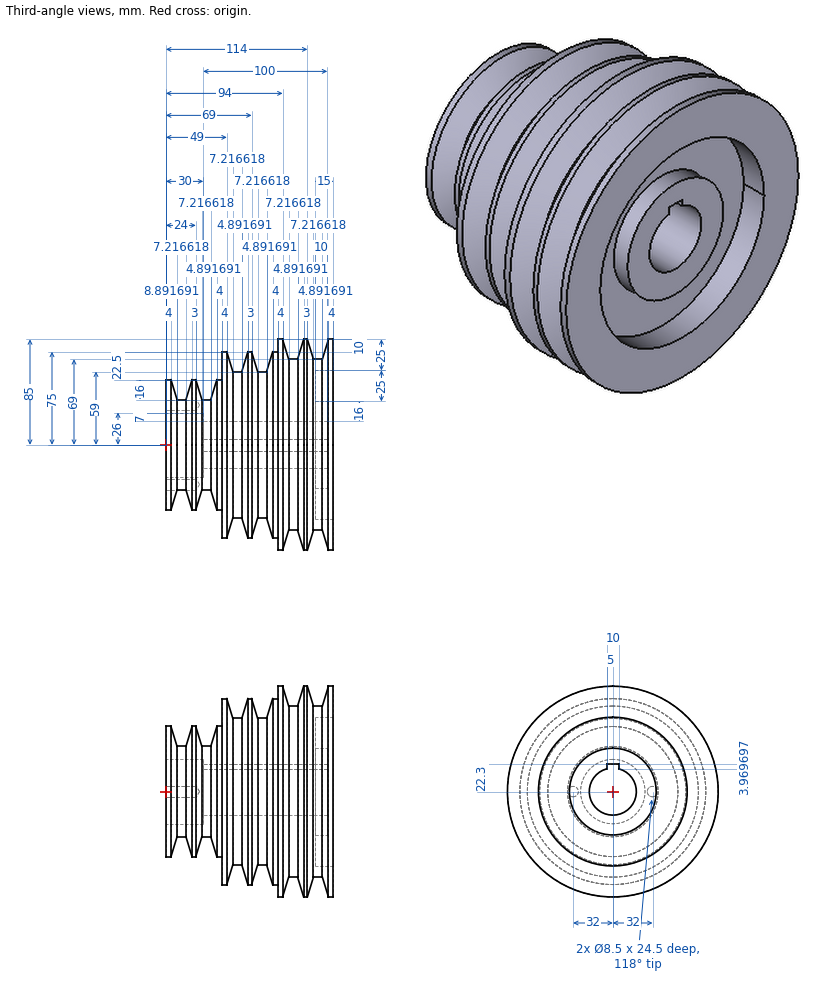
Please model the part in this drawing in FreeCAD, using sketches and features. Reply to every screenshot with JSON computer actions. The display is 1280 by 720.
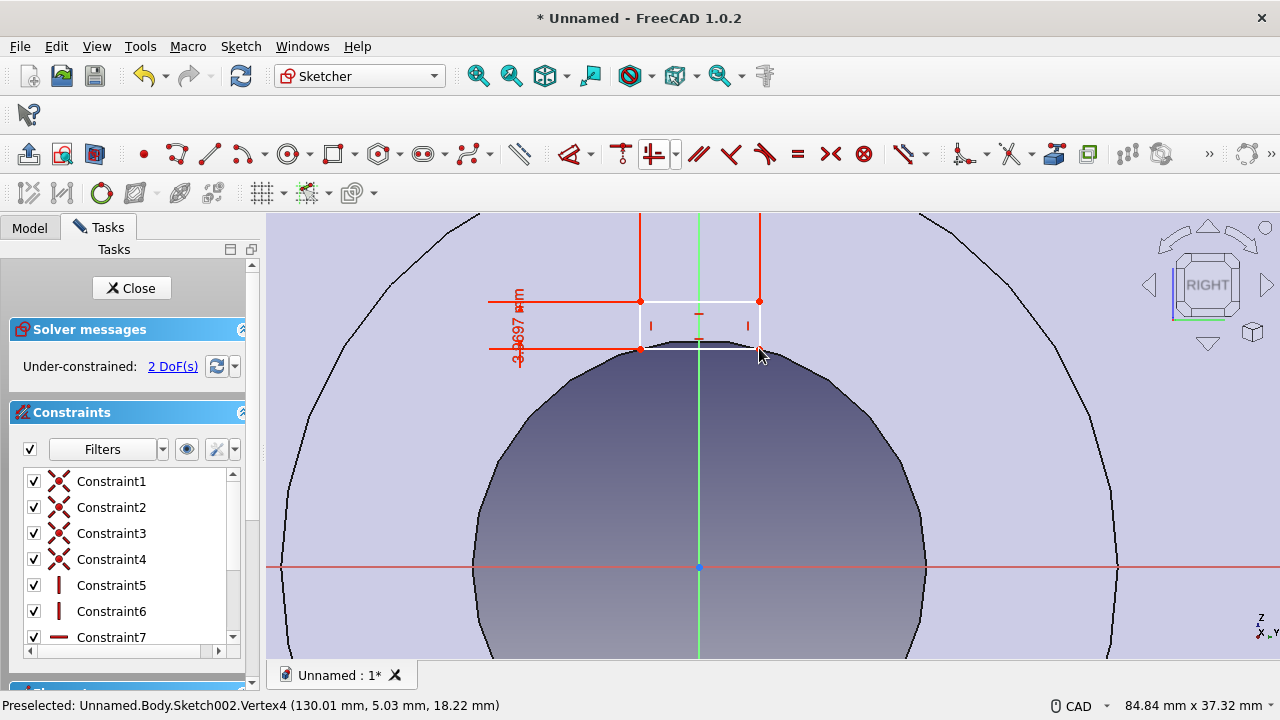
{"action": "left_click", "coordinate": [568, 154]}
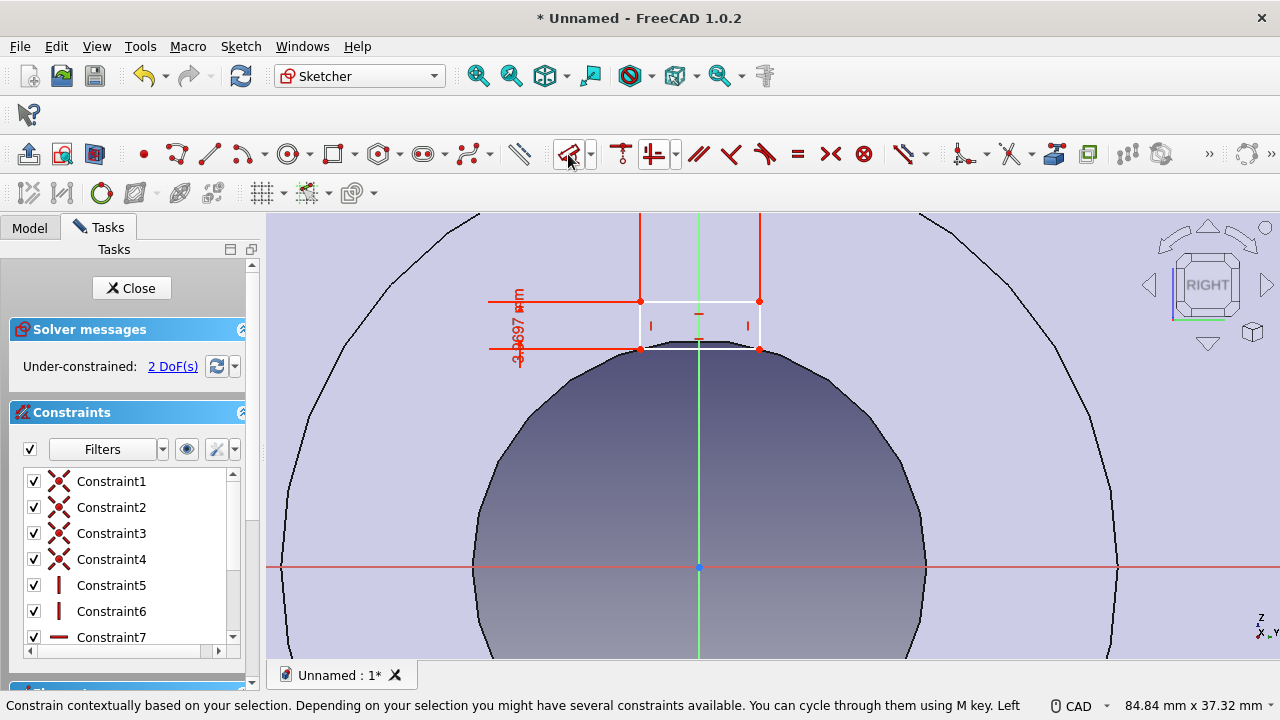
{"action": "left_click", "coordinate": [640, 302]}
{"action": "left_click", "coordinate": [670, 601]}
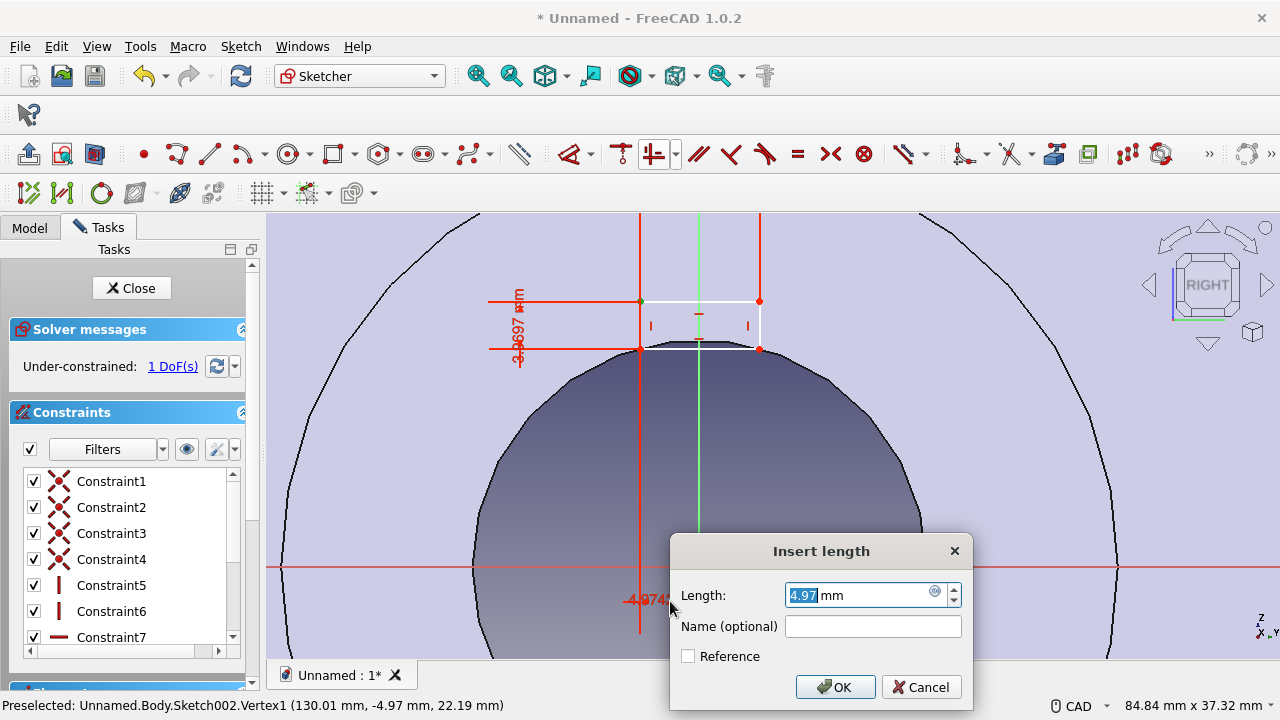
{"action": "type", "text": "5"}
{"action": "key", "text": "Return"}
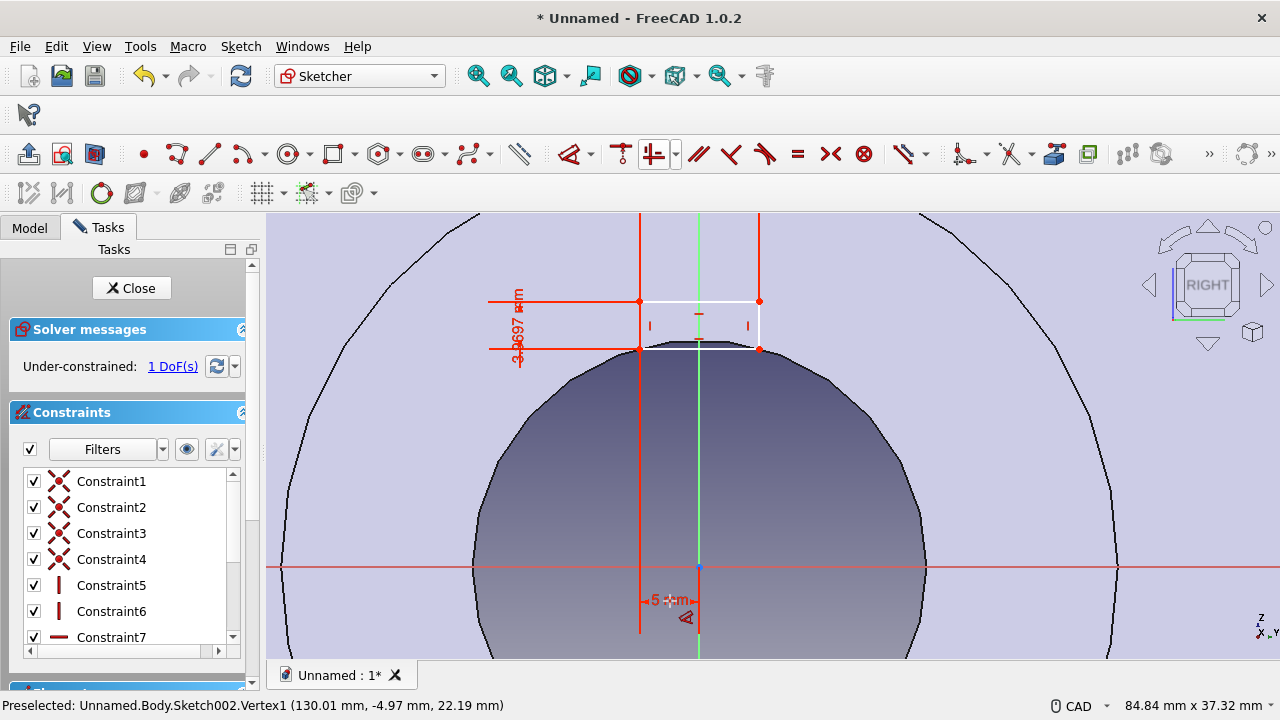
{"action": "left_click", "coordinate": [640, 302]}
{"action": "left_click", "coordinate": [606, 435]}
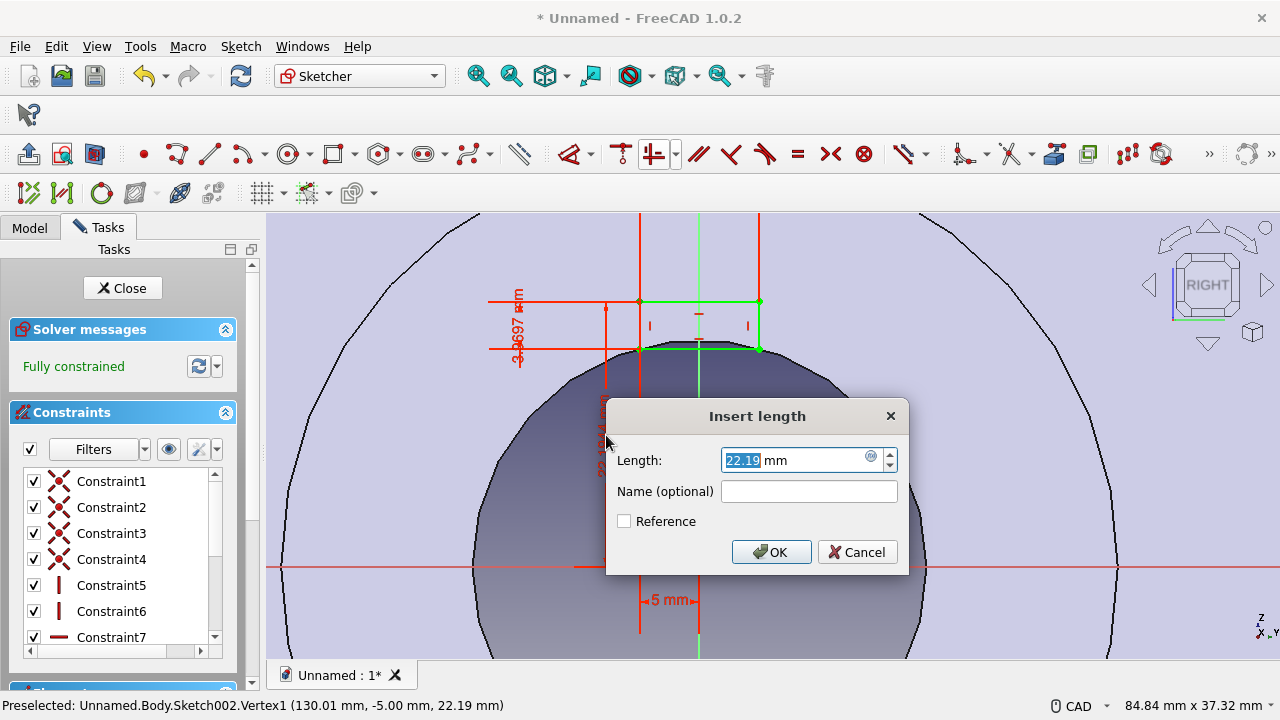
{"action": "type", "text": "22.3"}
{"action": "key", "text": "Return"}
{"action": "key", "text": "Escape"}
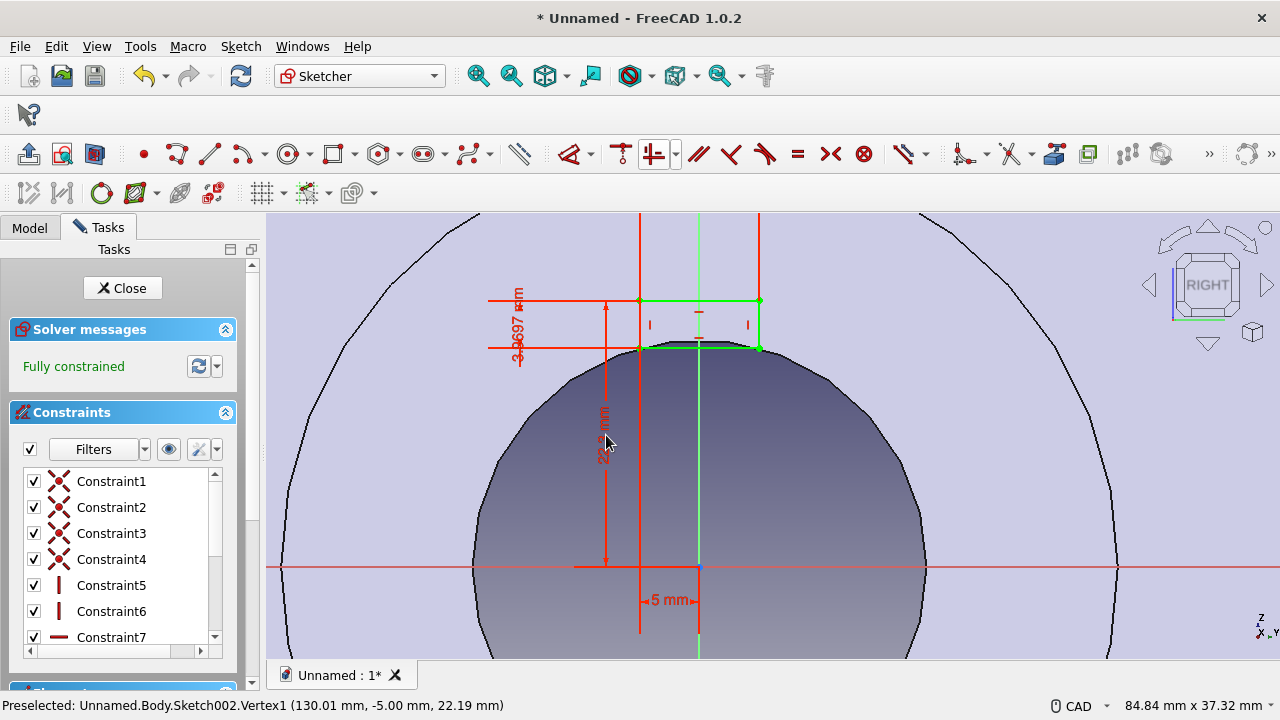
{"action": "left_click", "coordinate": [123, 288]}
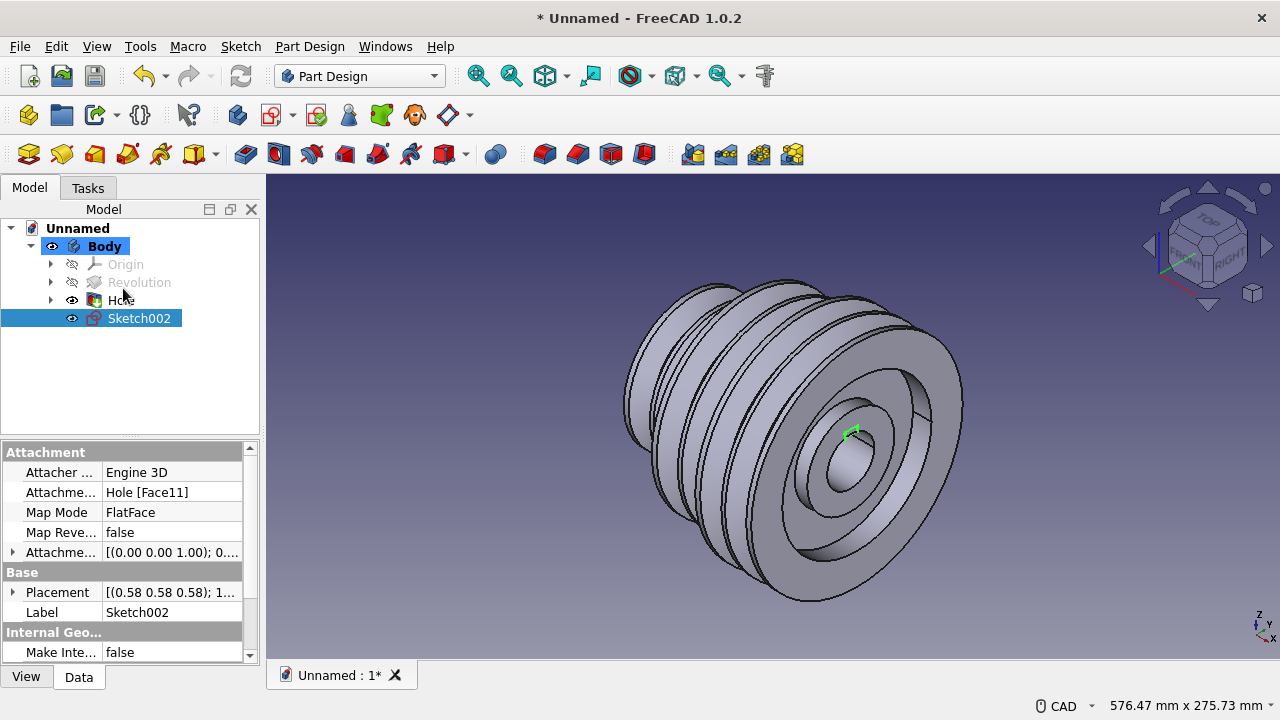
{"action": "left_click", "coordinate": [246, 154]}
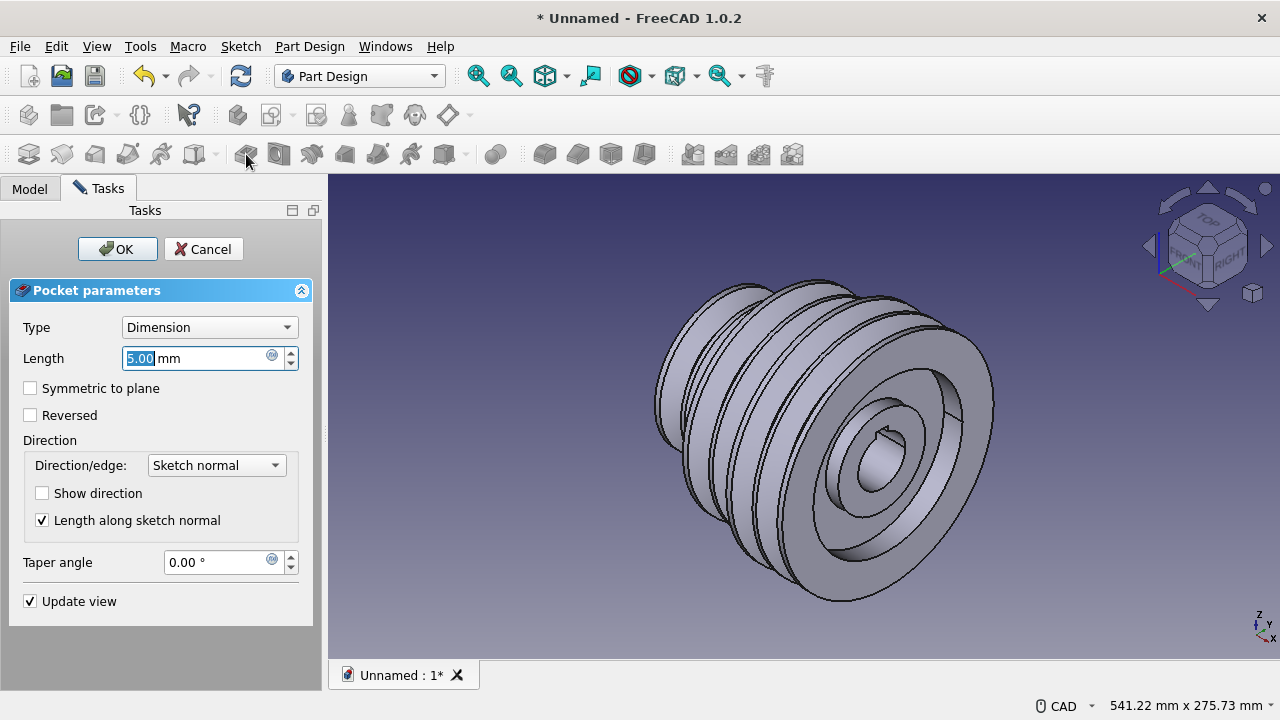
{"action": "left_click", "coordinate": [210, 328]}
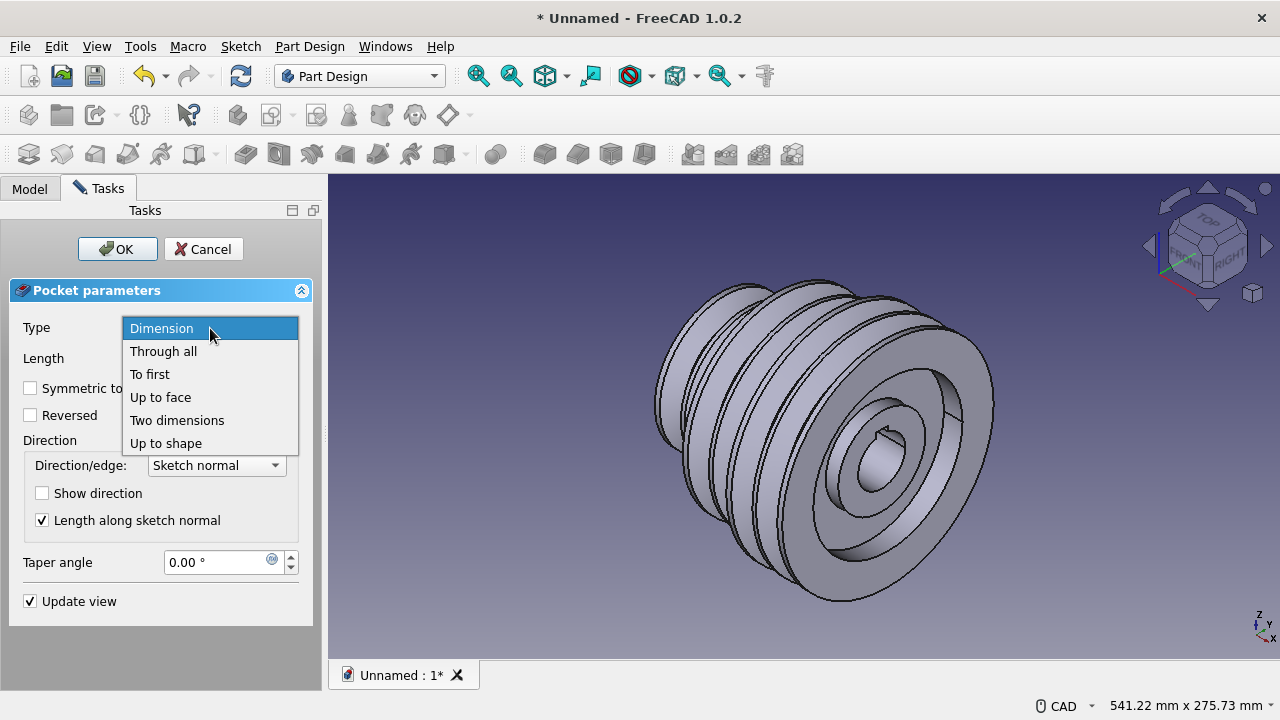
{"action": "left_click", "coordinate": [208, 352]}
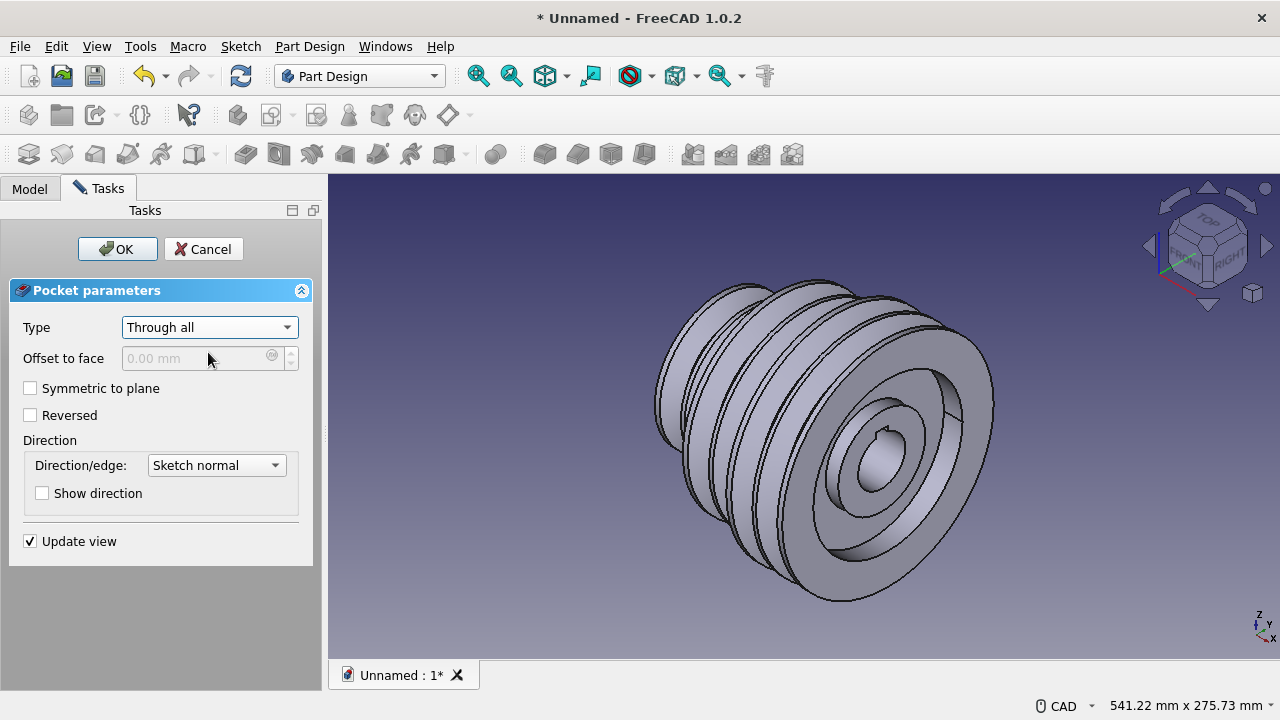
{"action": "left_click", "coordinate": [118, 249]}